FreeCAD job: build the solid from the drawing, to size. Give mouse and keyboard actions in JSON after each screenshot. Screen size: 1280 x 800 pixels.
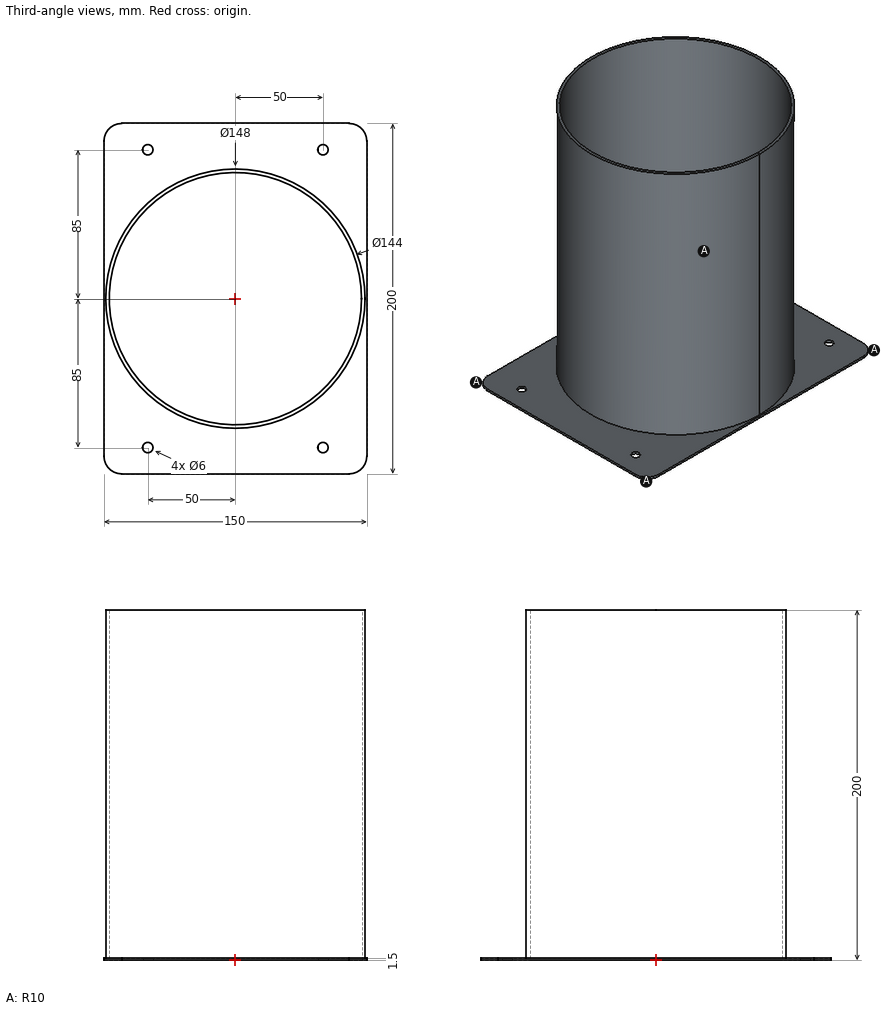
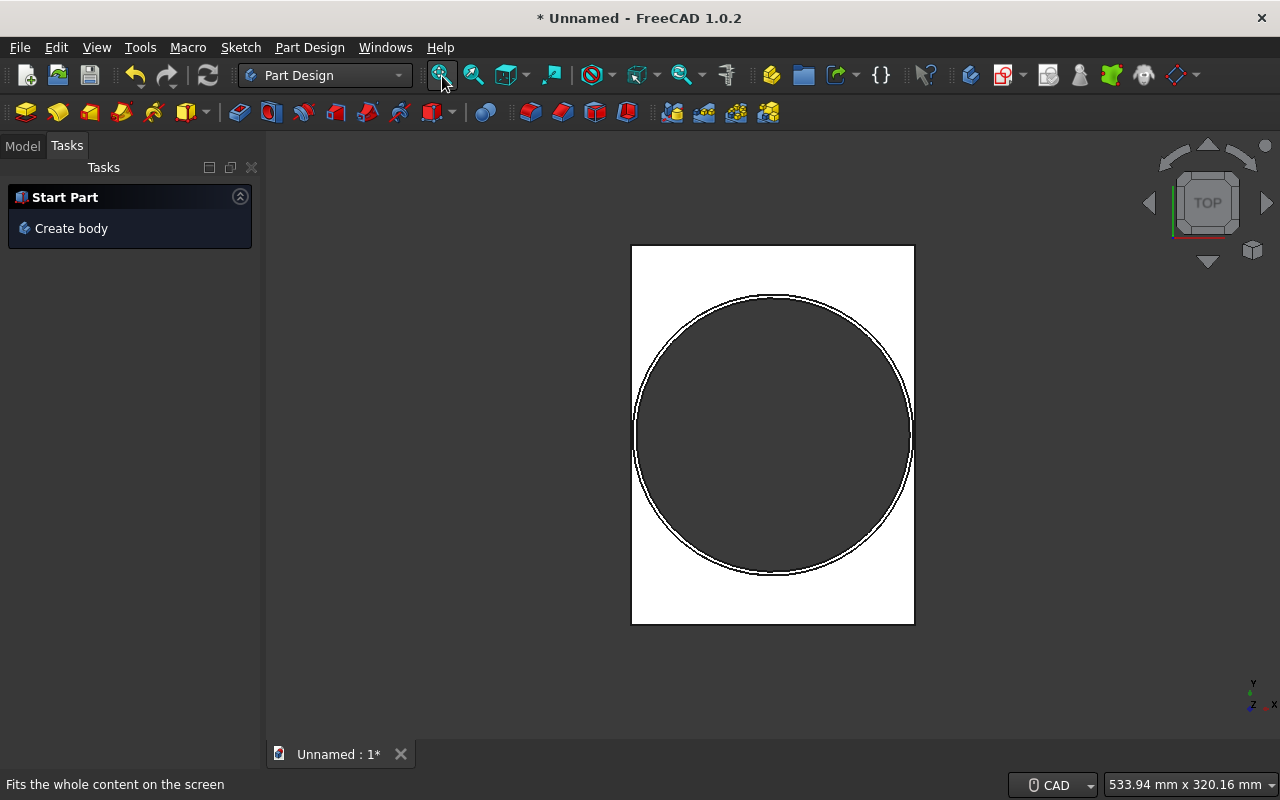
{"action": "key", "text": "1"}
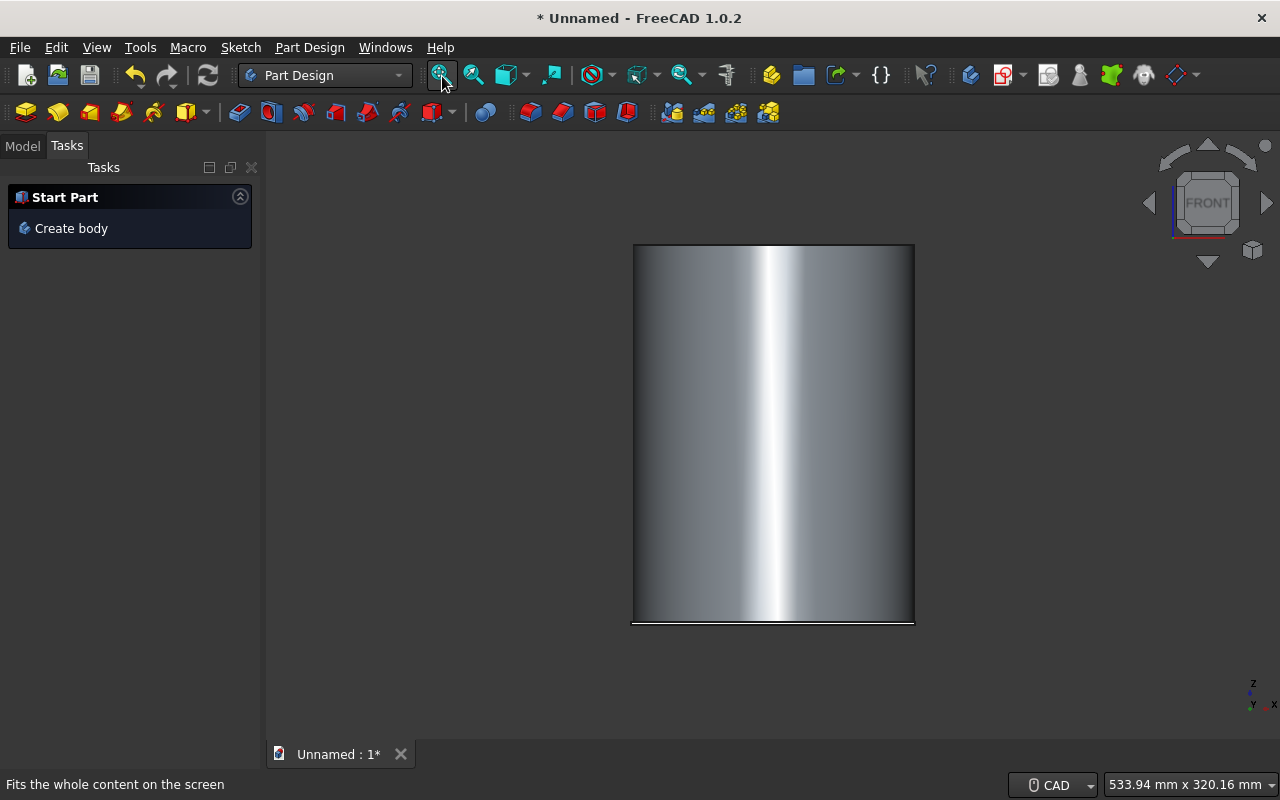
{"action": "scroll", "coordinate": [631, 622], "scroll_direction": "up", "scroll_amount": 14}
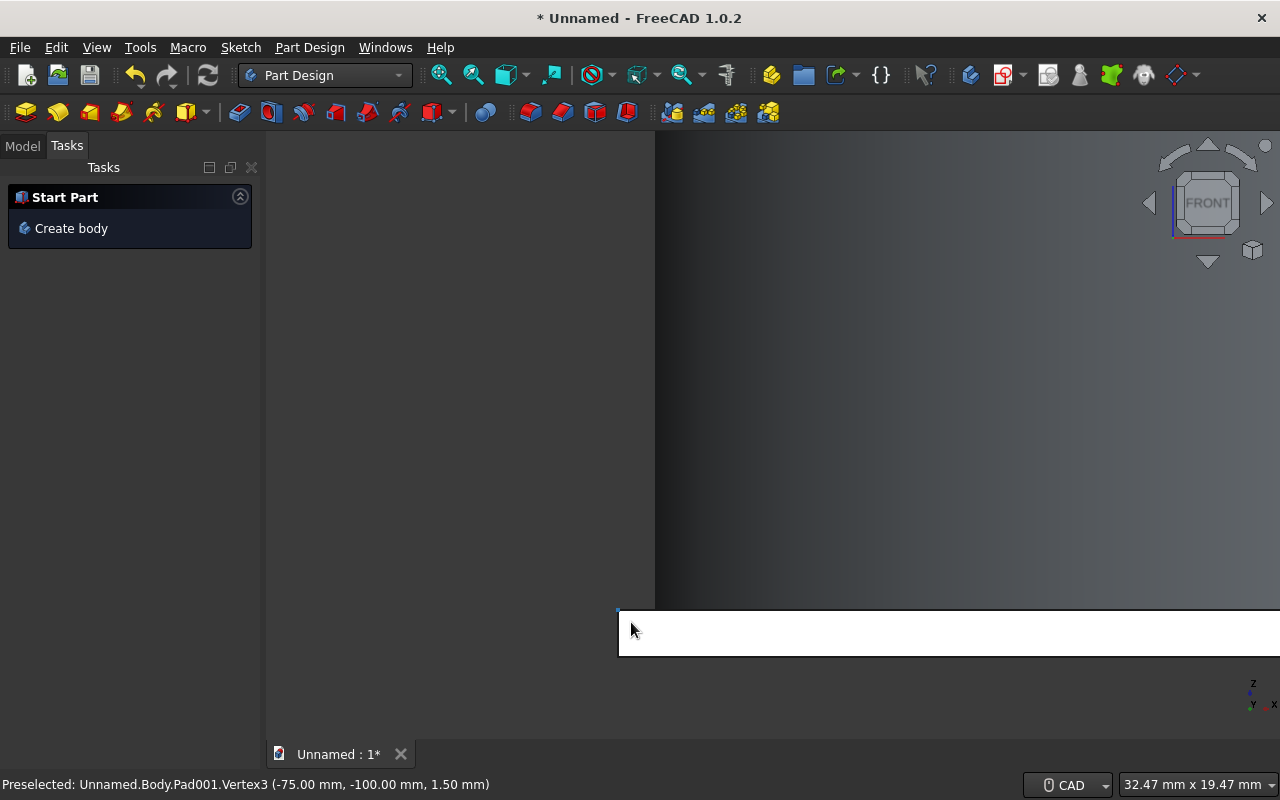
{"action": "left_click", "coordinate": [618, 633]}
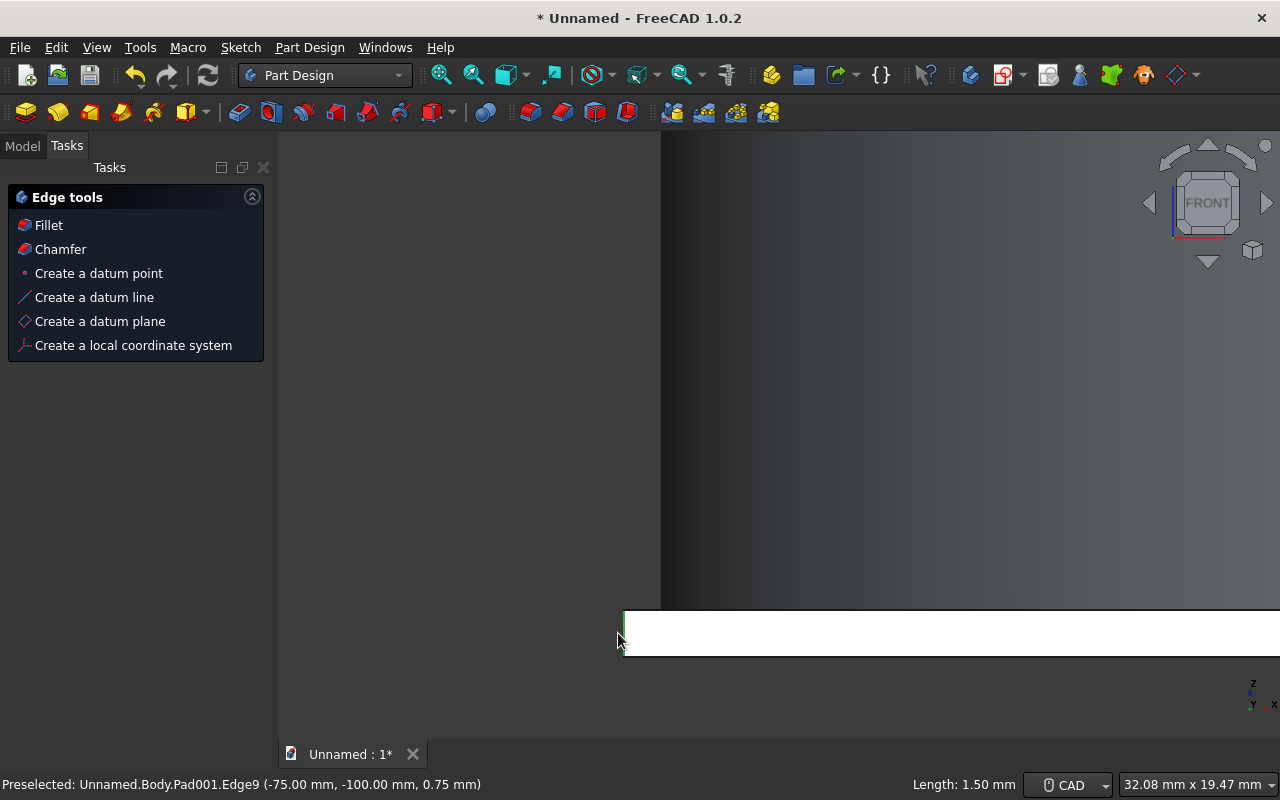
{"action": "left_click", "coordinate": [442, 76]}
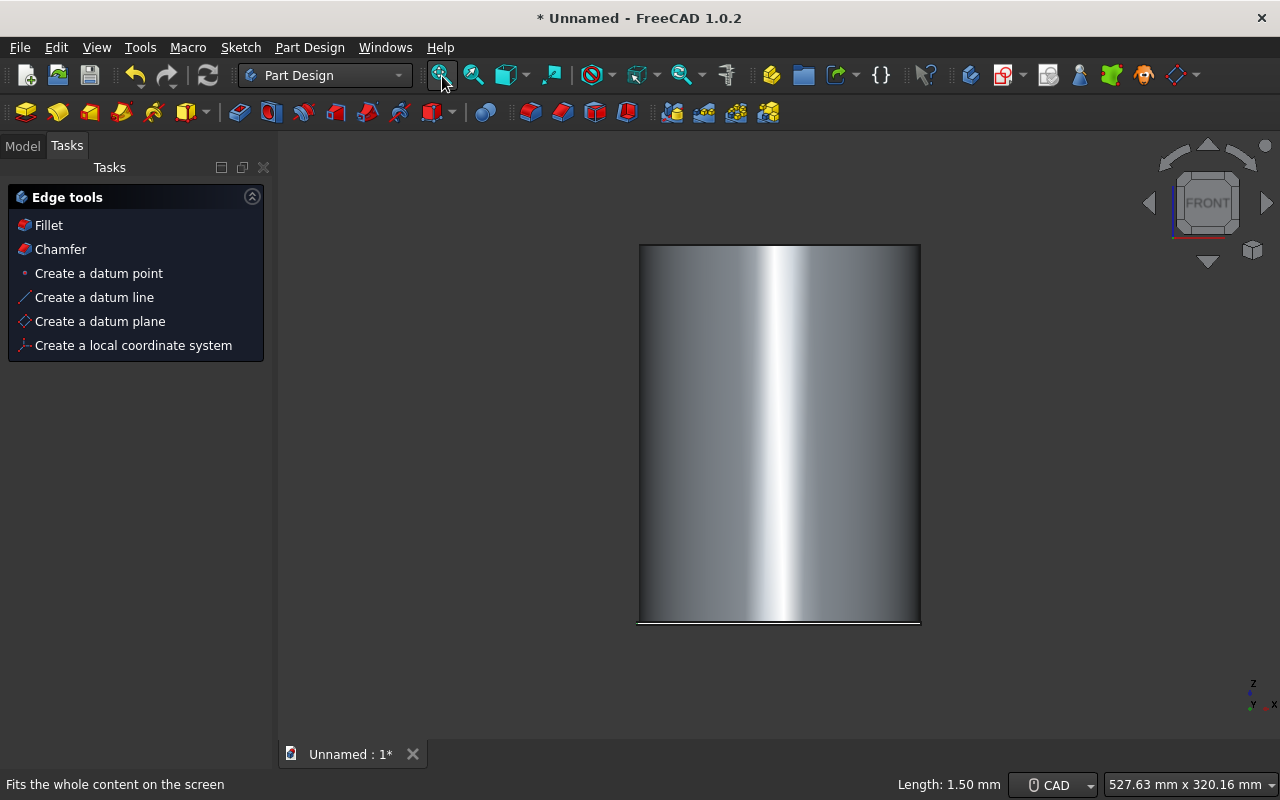
{"action": "key", "text": "3"}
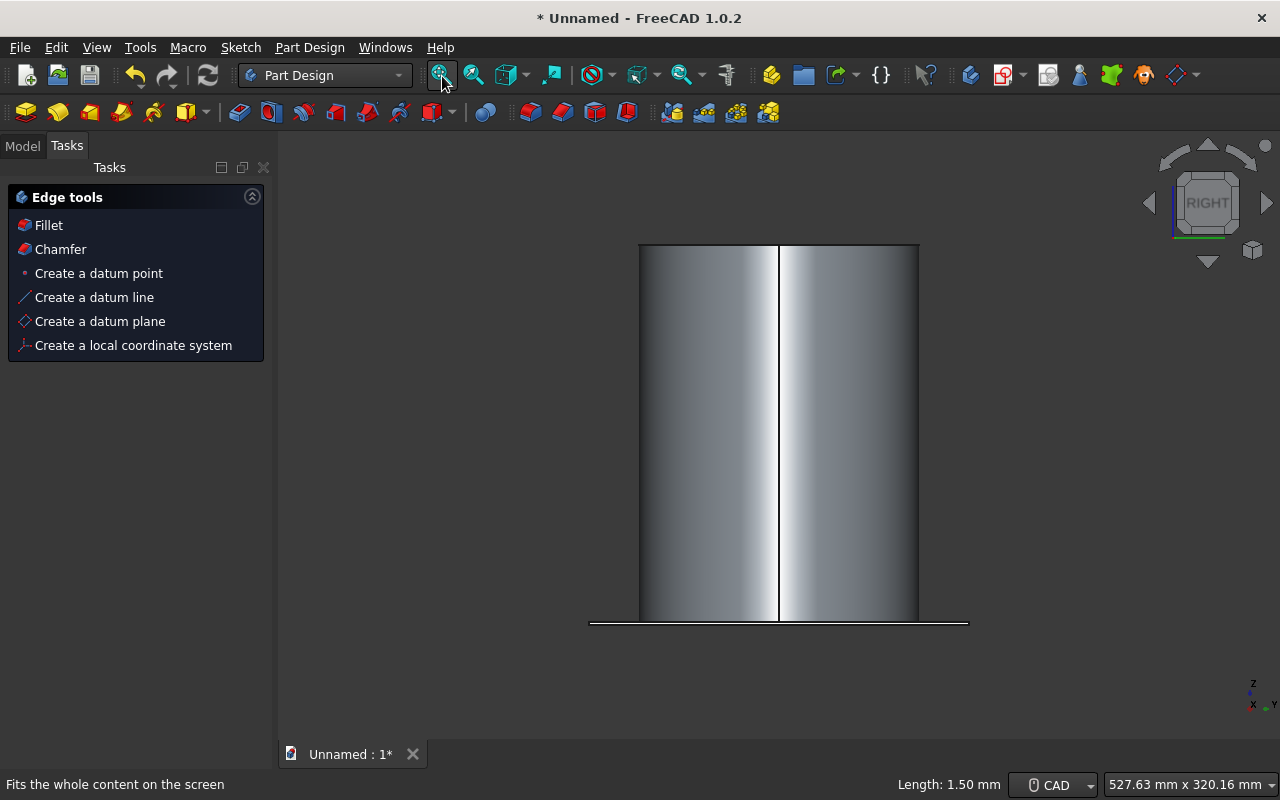
{"action": "scroll", "coordinate": [969, 622], "scroll_direction": "up", "scroll_amount": 14}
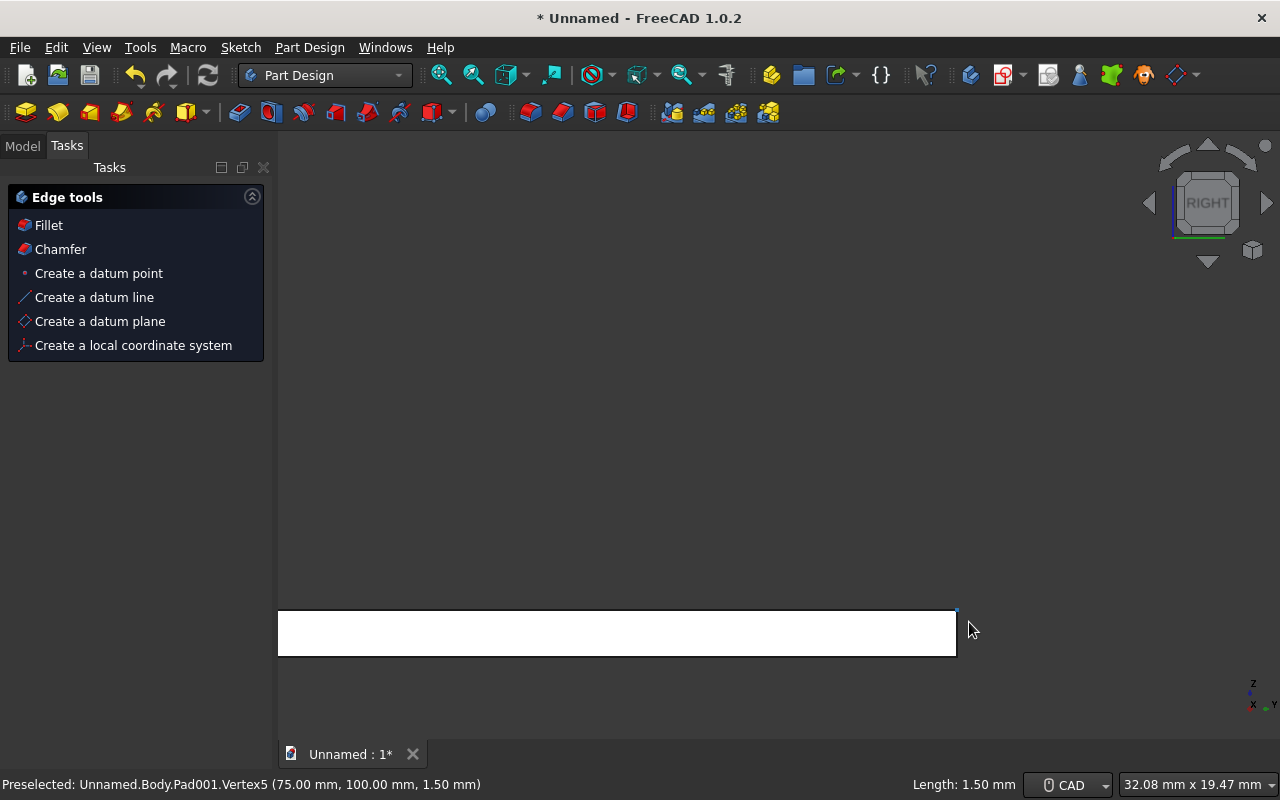
{"action": "left_click", "coordinate": [957, 633], "text": "ctrl"}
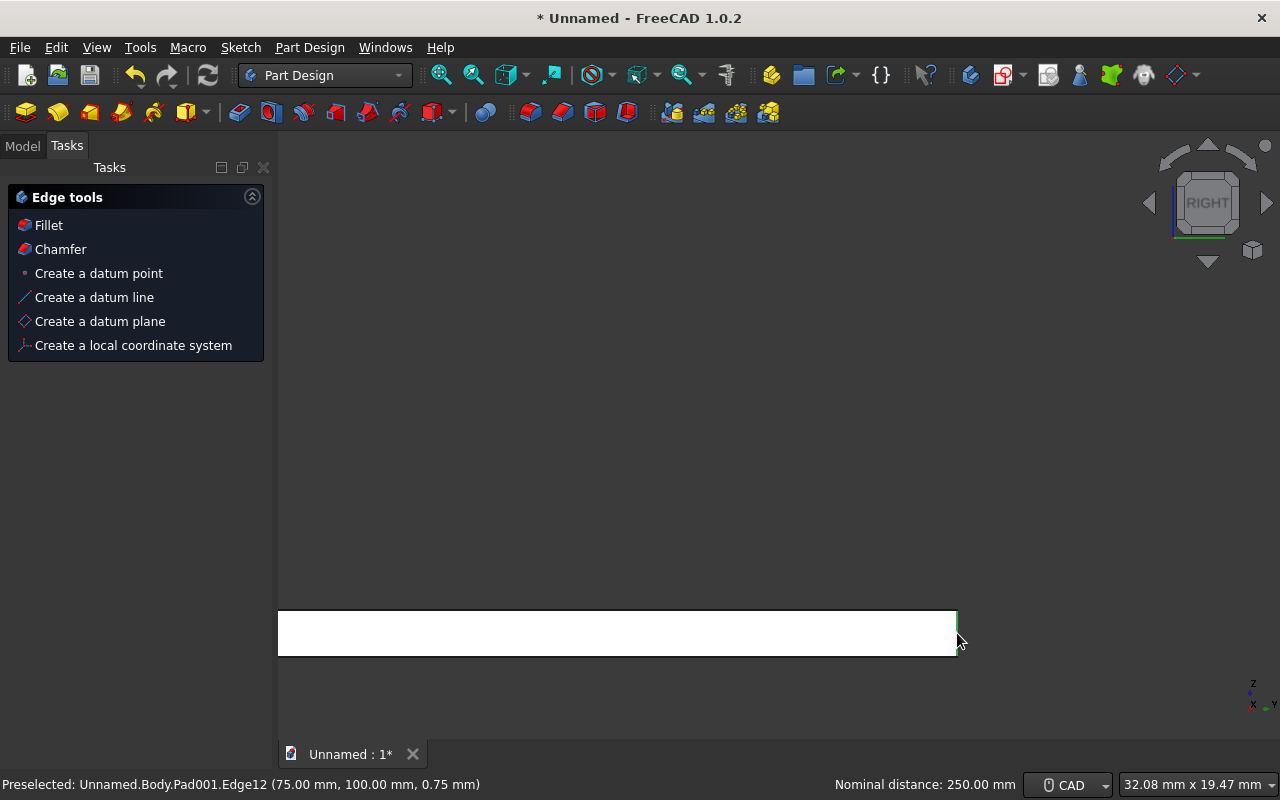
{"action": "left_click", "coordinate": [442, 76]}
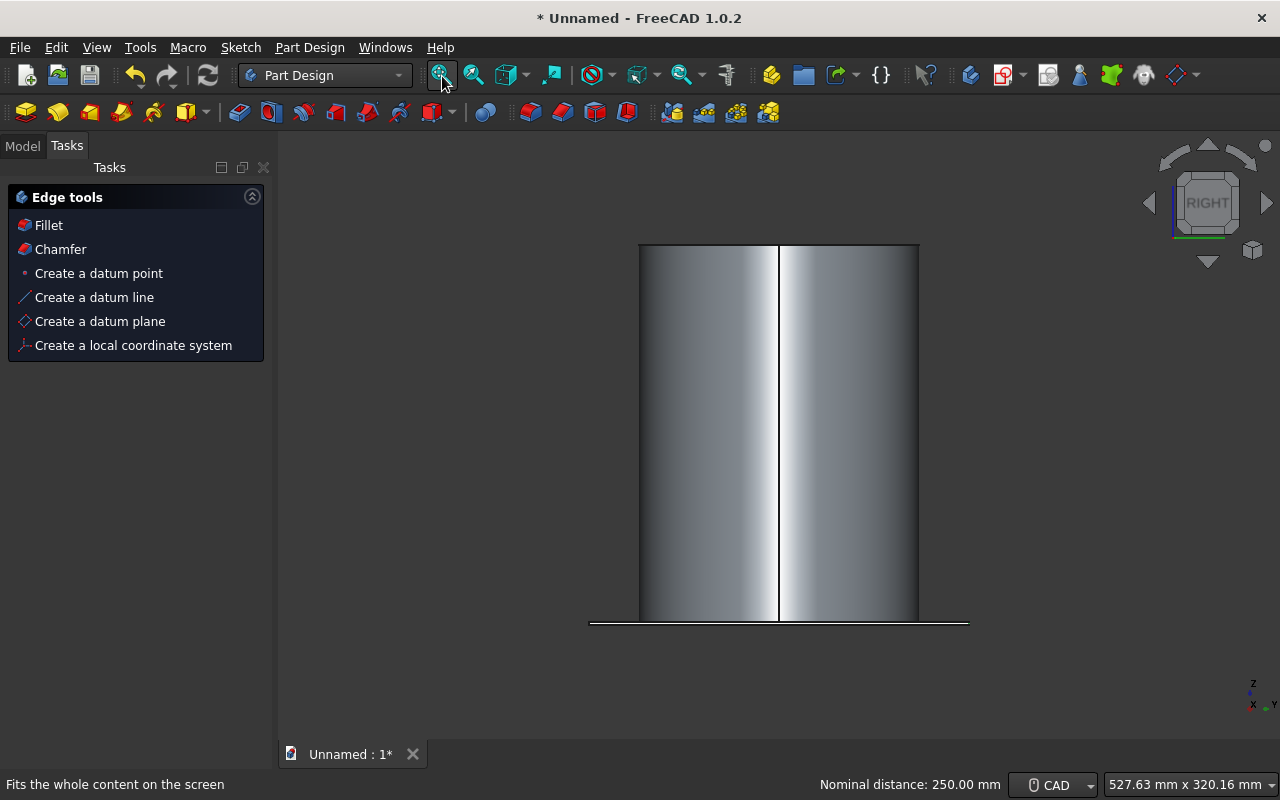
{"action": "key", "text": "5"}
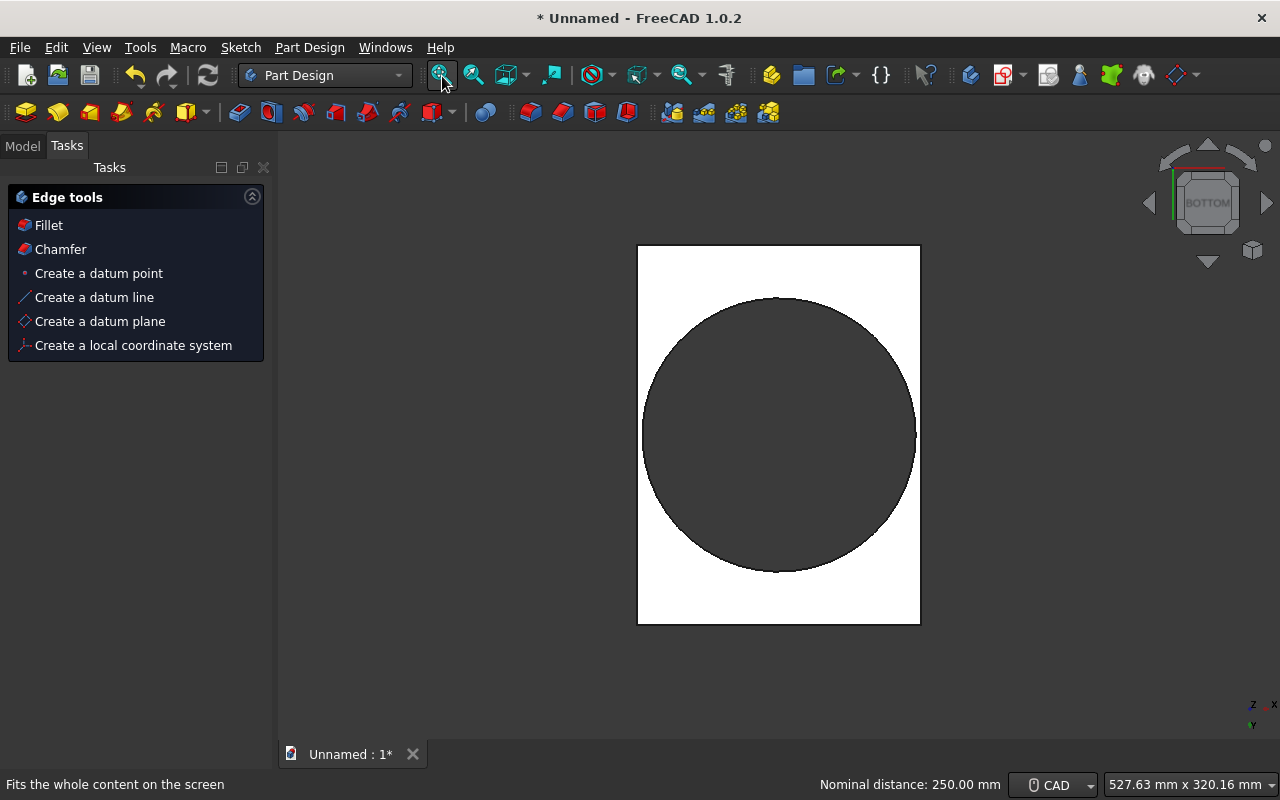
{"action": "scroll", "coordinate": [637, 624], "scroll_direction": "up", "scroll_amount": 14}